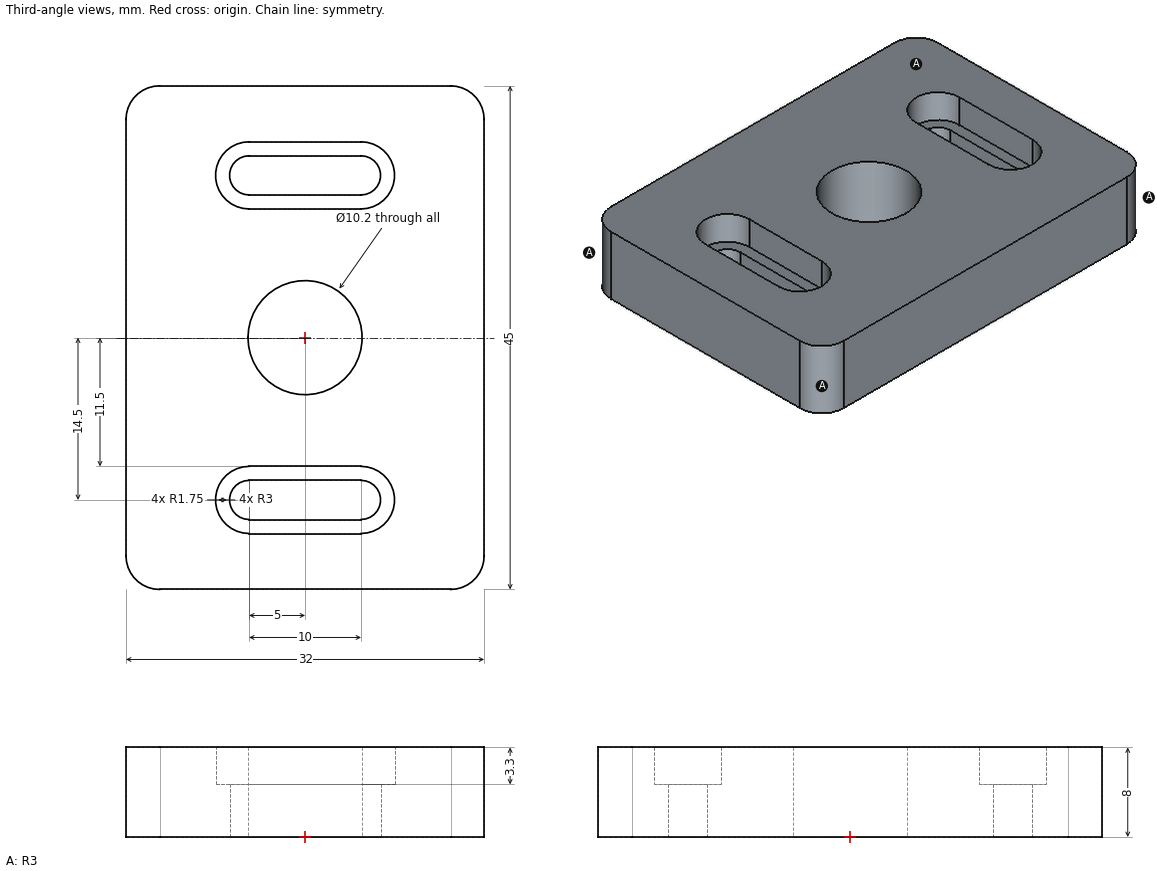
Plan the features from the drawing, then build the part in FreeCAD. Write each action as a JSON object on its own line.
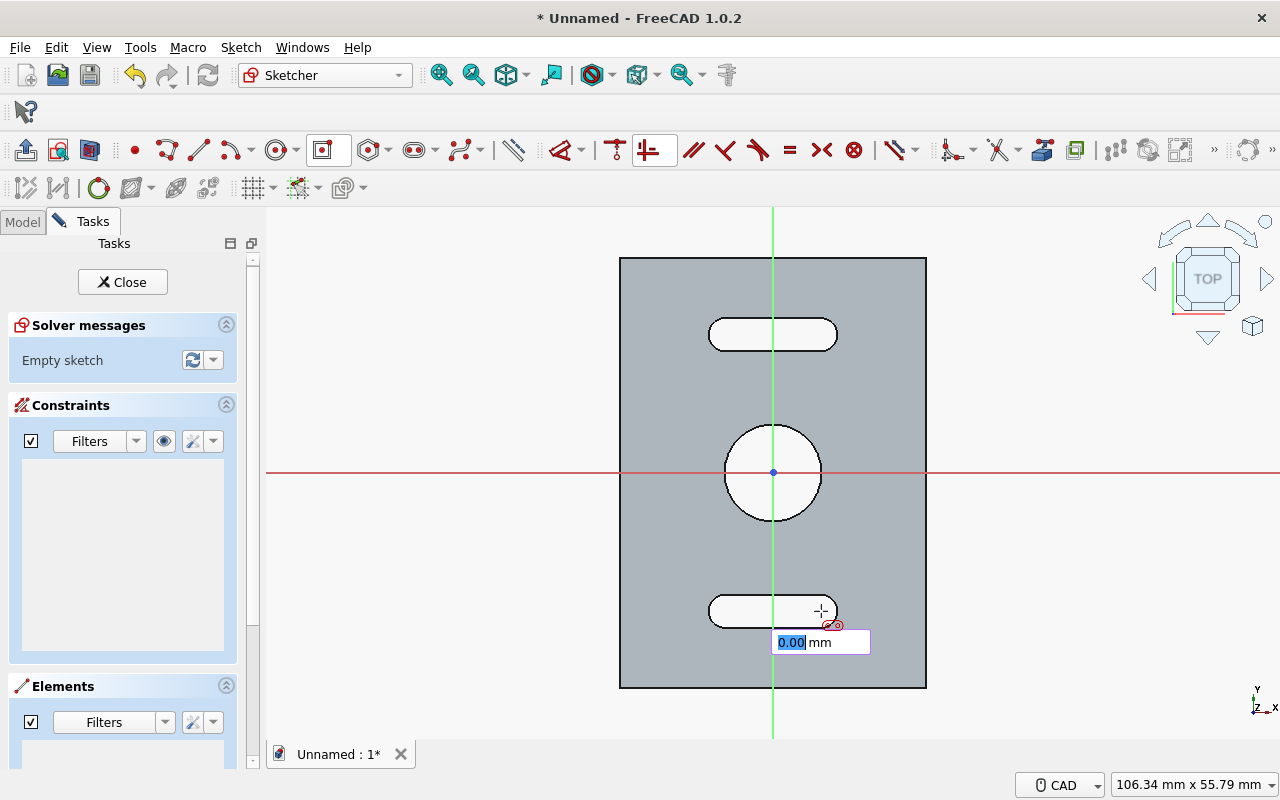
{"action": "left_click", "coordinate": [787, 583]}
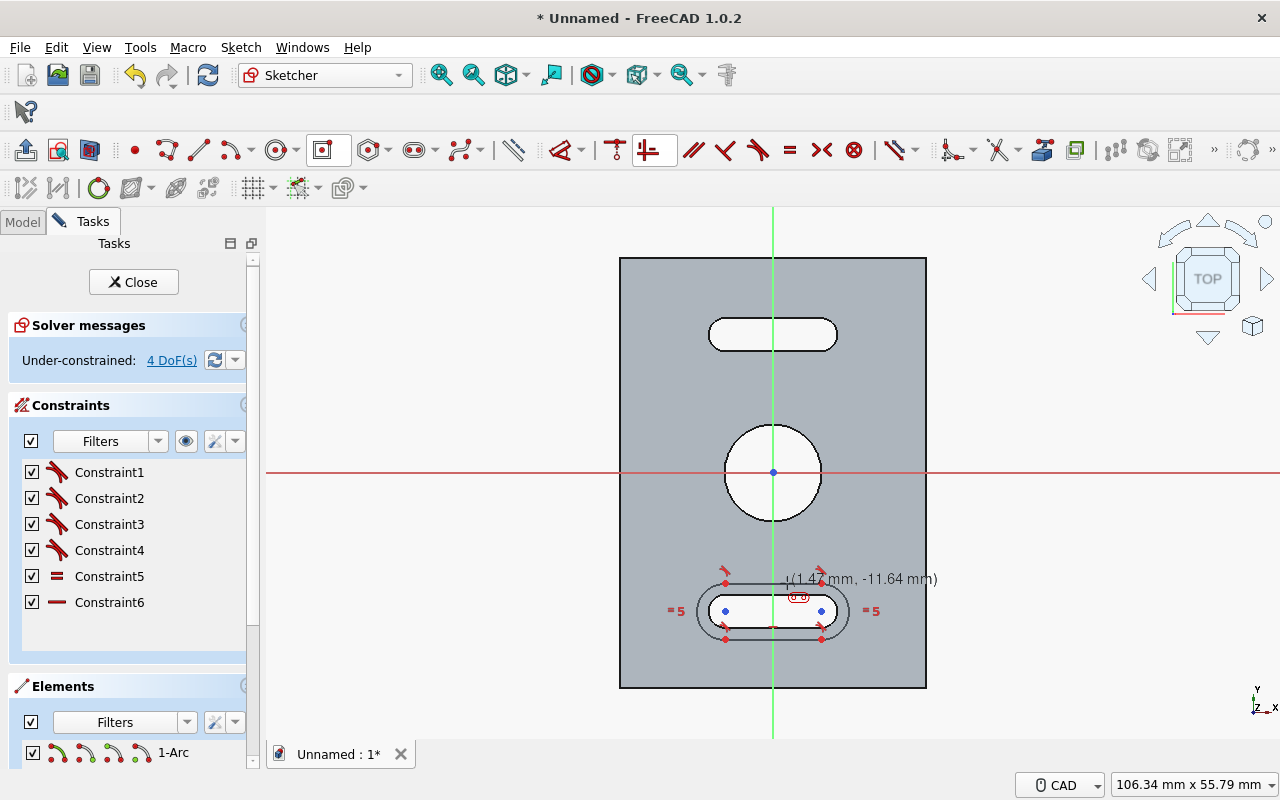
{"action": "left_click", "coordinate": [725, 335]}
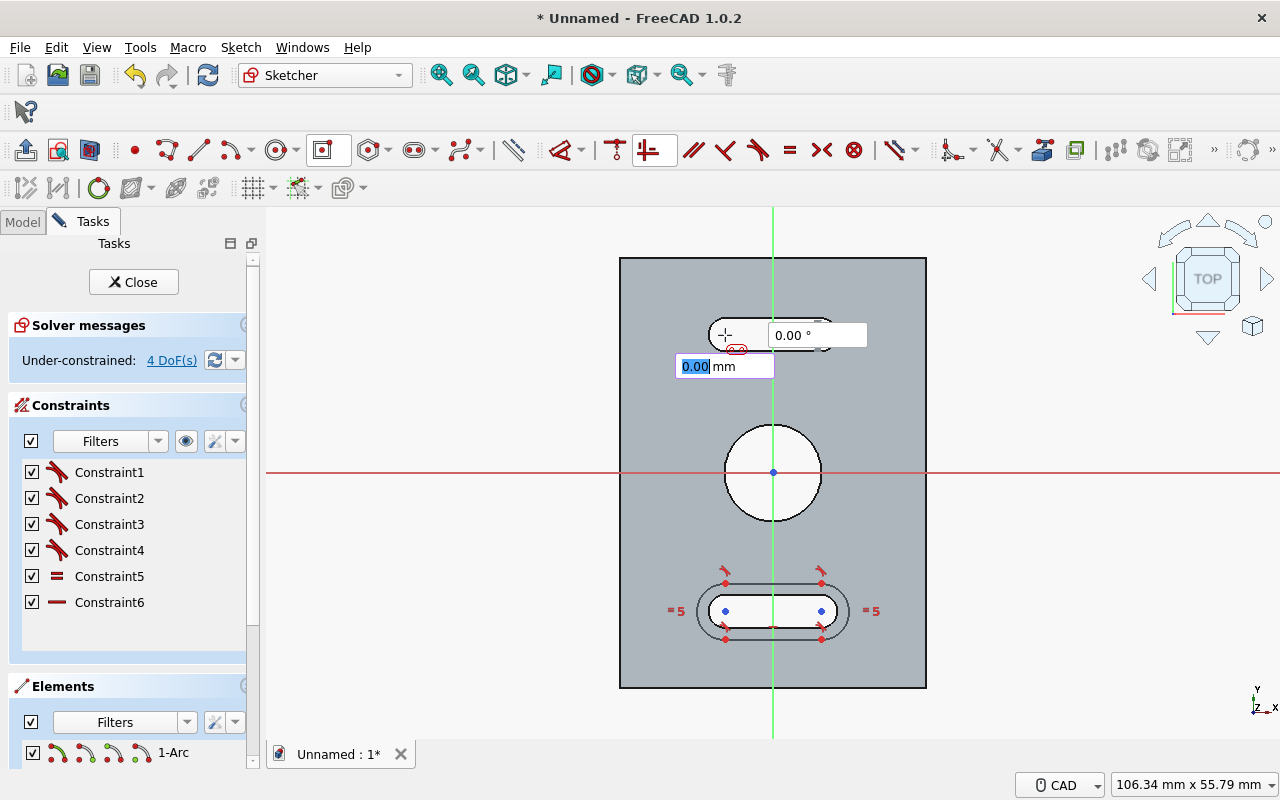
{"action": "left_click", "coordinate": [821, 335]}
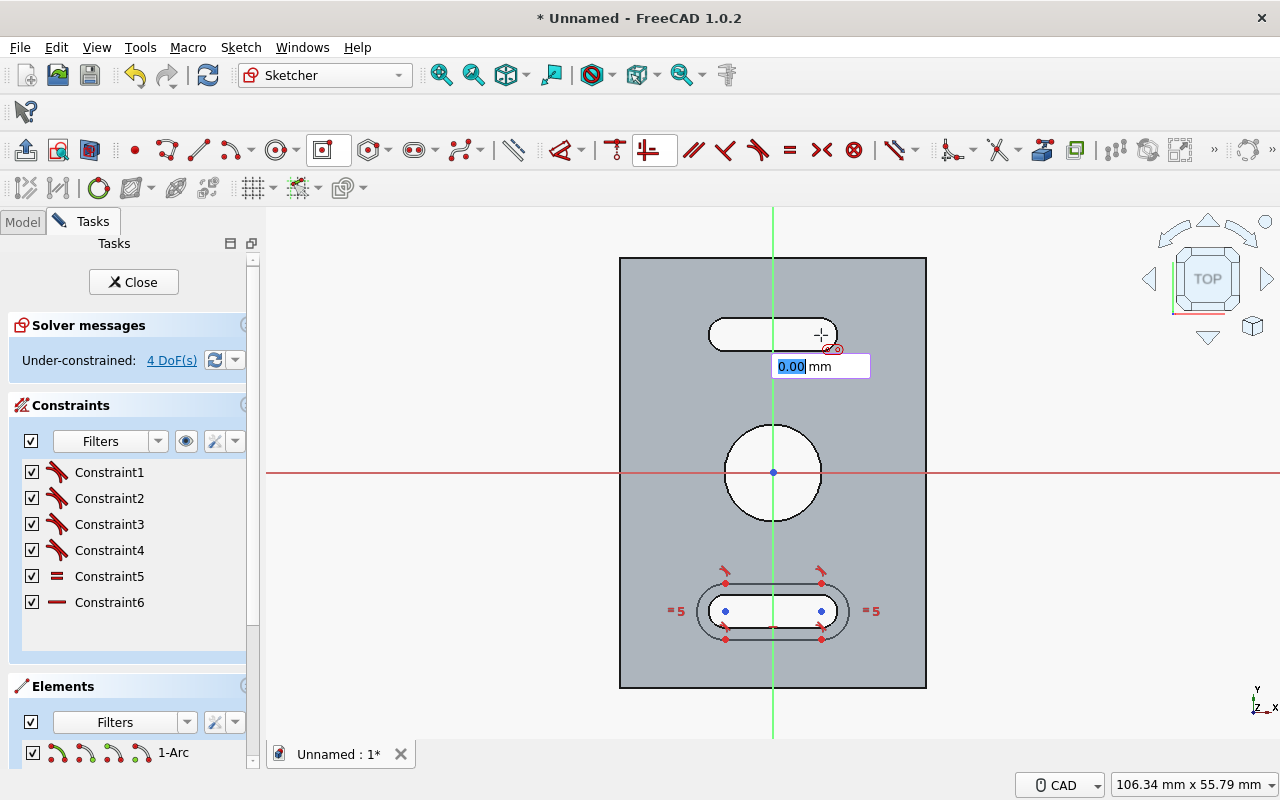
{"action": "left_click", "coordinate": [787, 306]}
{"action": "key", "text": "Escape"}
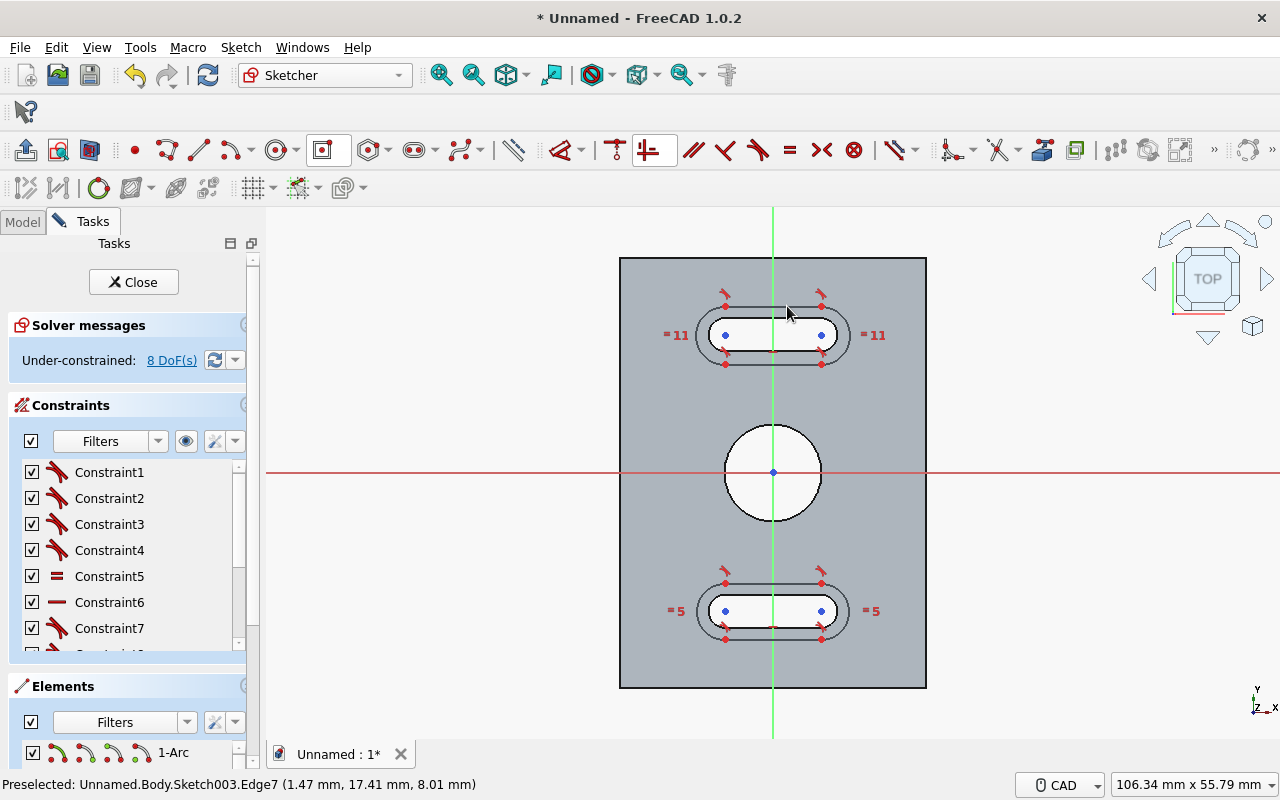
{"action": "left_click", "coordinate": [702, 596]}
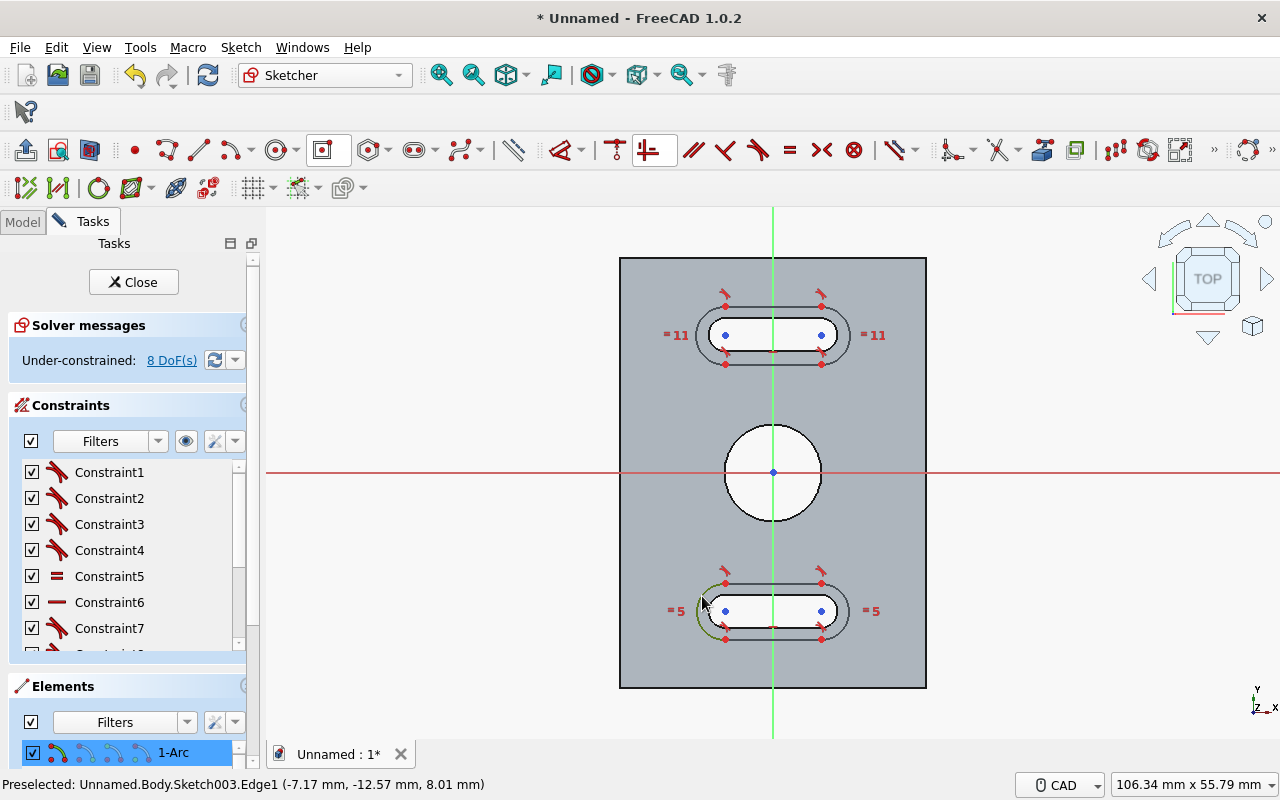
{"action": "left_click", "coordinate": [702, 319]}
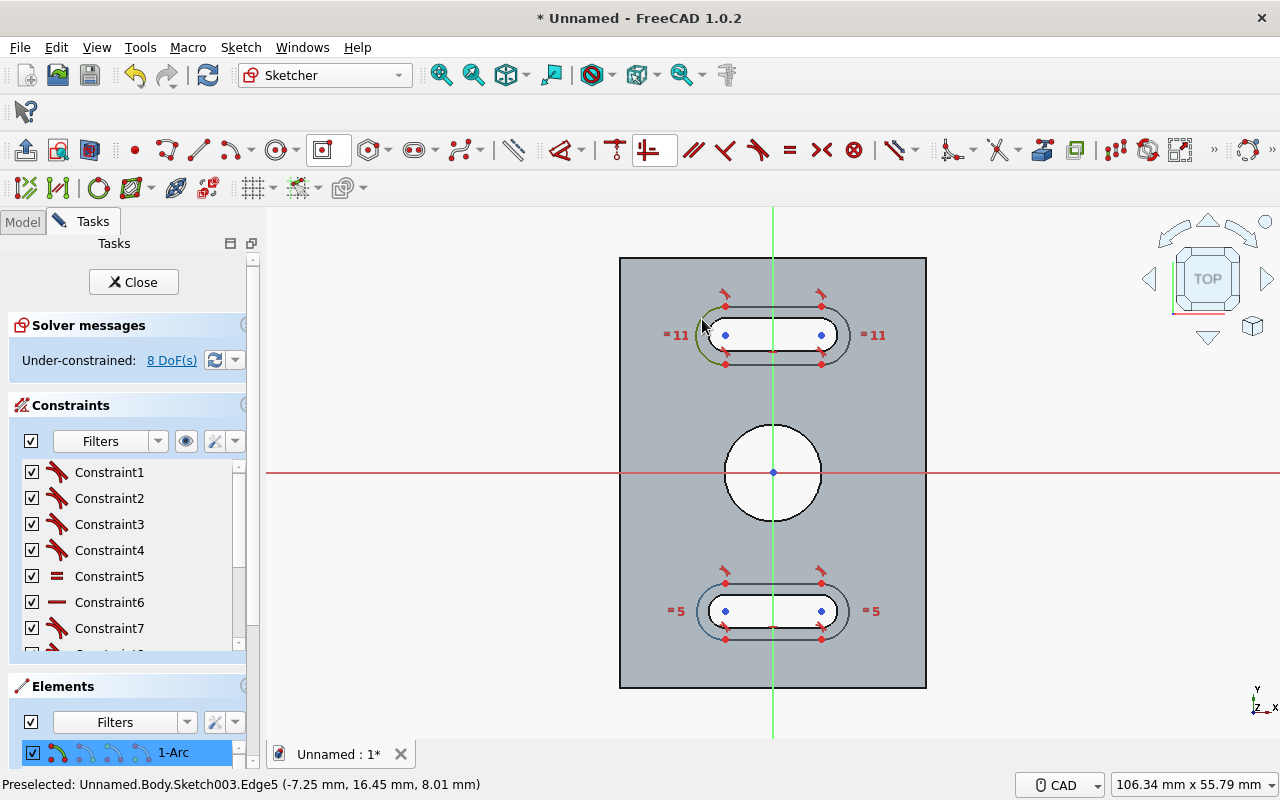
{"action": "left_click", "coordinate": [790, 150]}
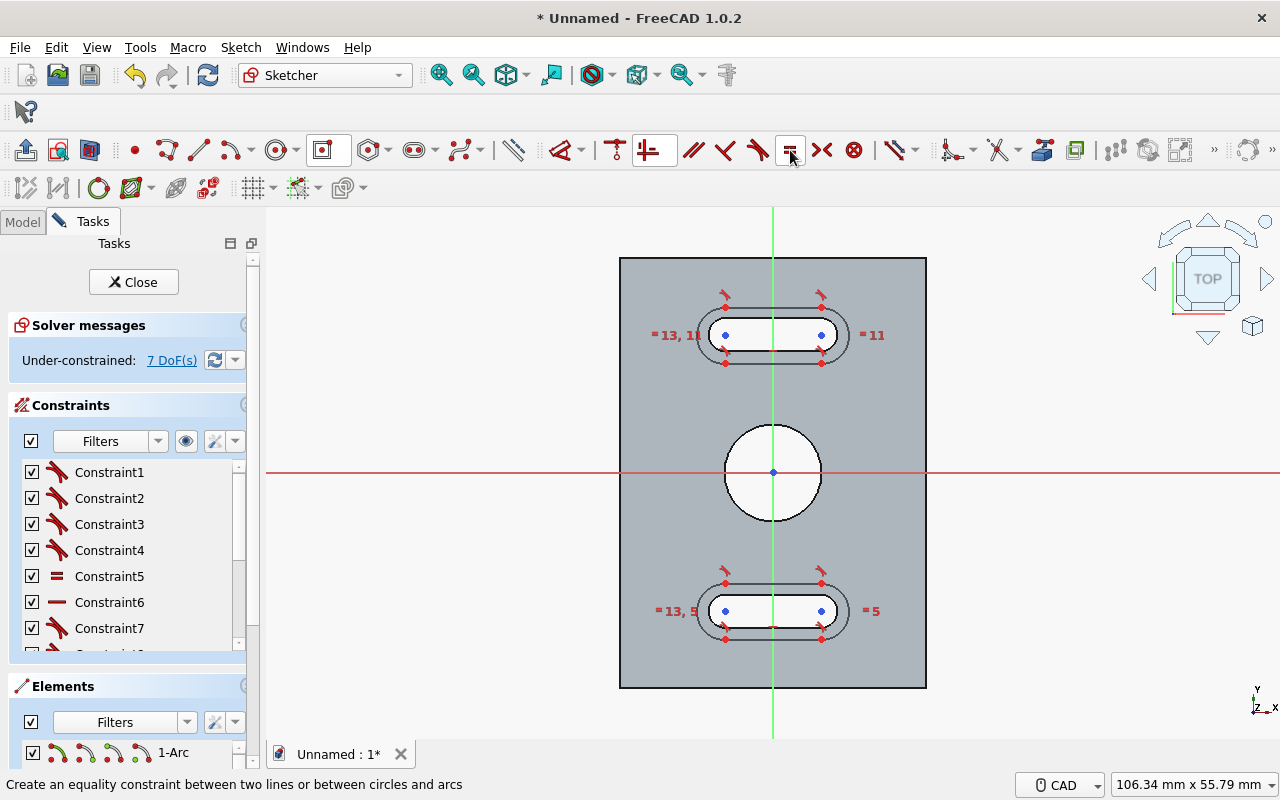
{"action": "left_click", "coordinate": [725, 612]}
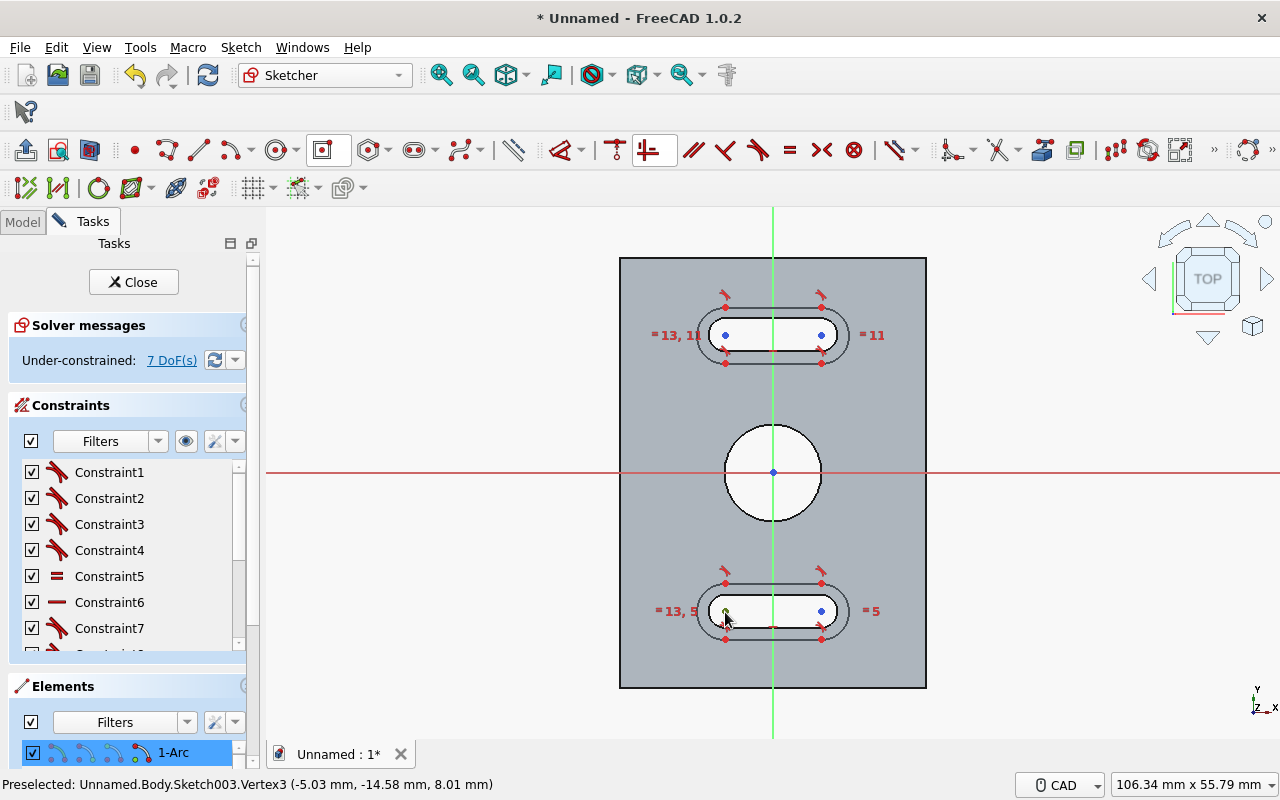
{"action": "left_click", "coordinate": [725, 336]}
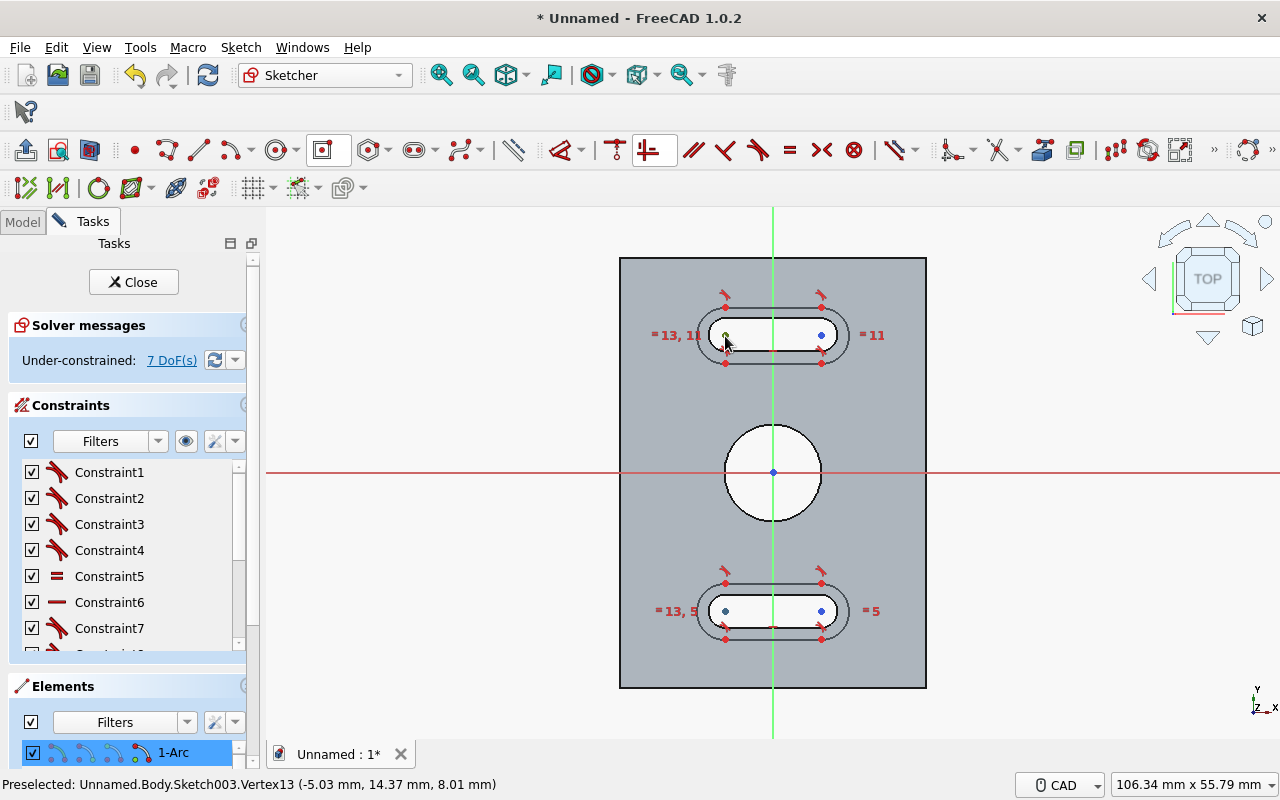
{"action": "left_click", "coordinate": [353, 473]}